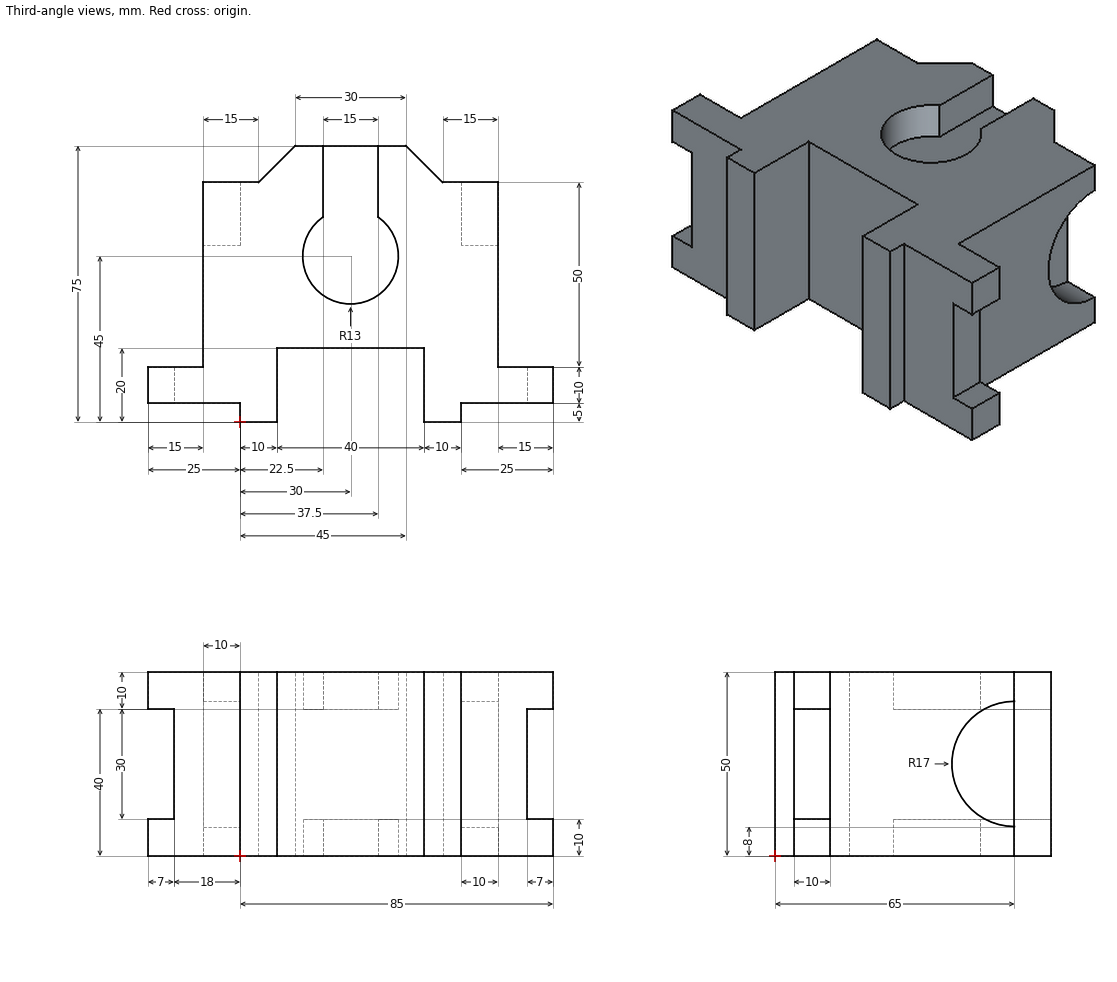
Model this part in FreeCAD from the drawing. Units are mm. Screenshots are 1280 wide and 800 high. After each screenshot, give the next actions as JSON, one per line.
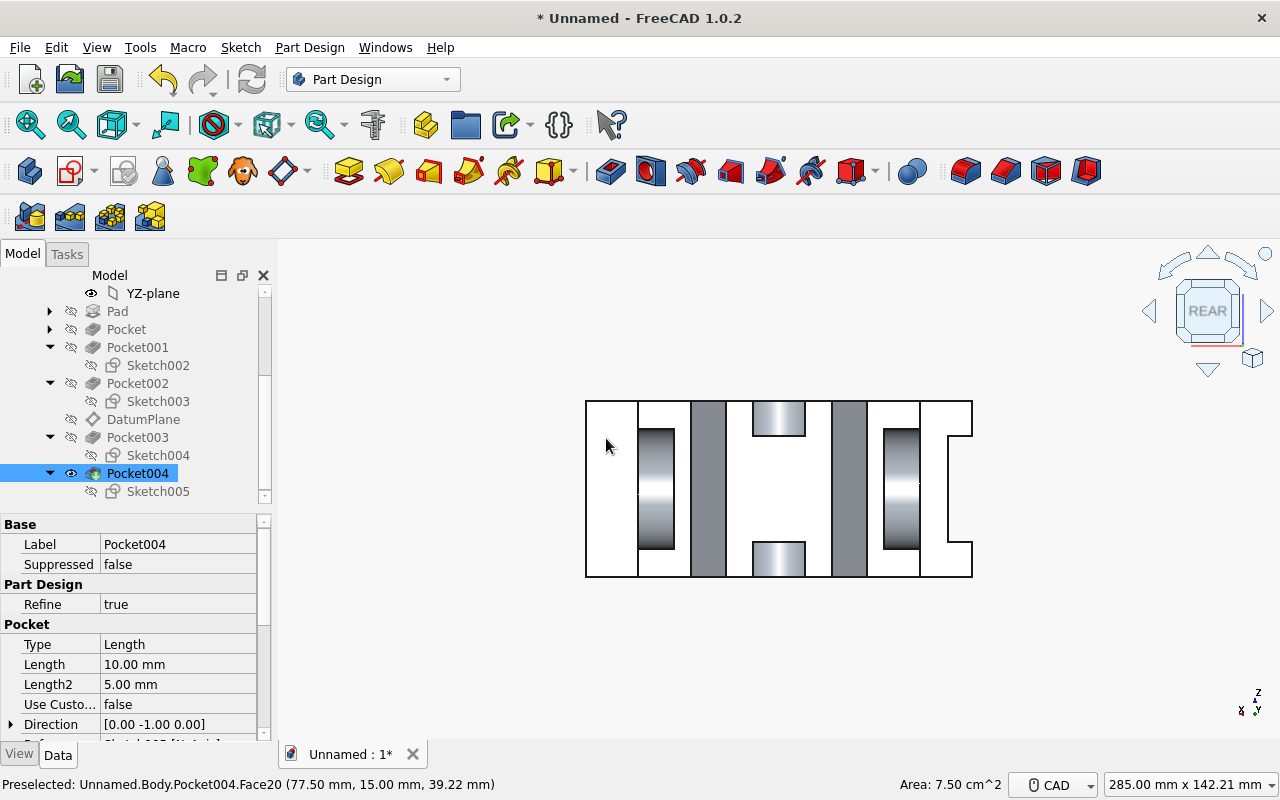
{"action": "left_click", "coordinate": [70, 172]}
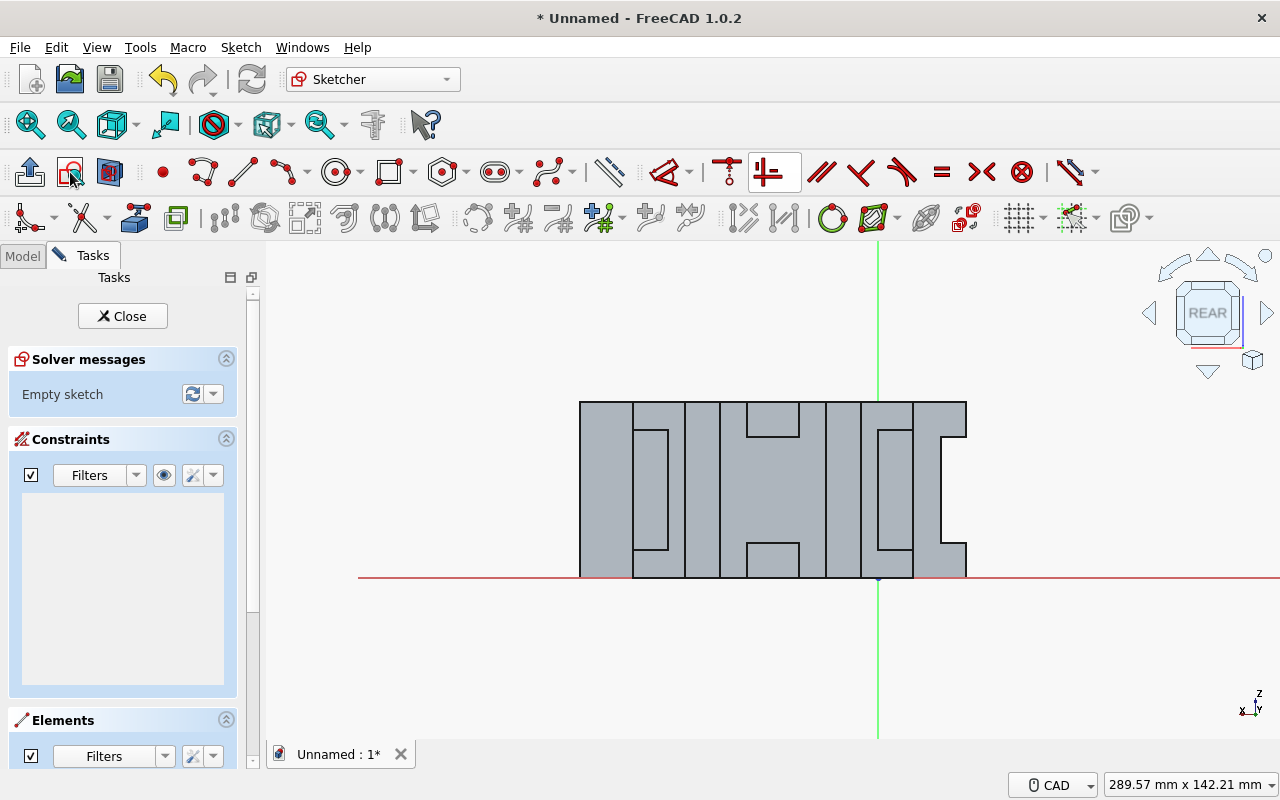
{"action": "scroll", "coordinate": [528, 490], "scroll_direction": "up", "scroll_amount": 5}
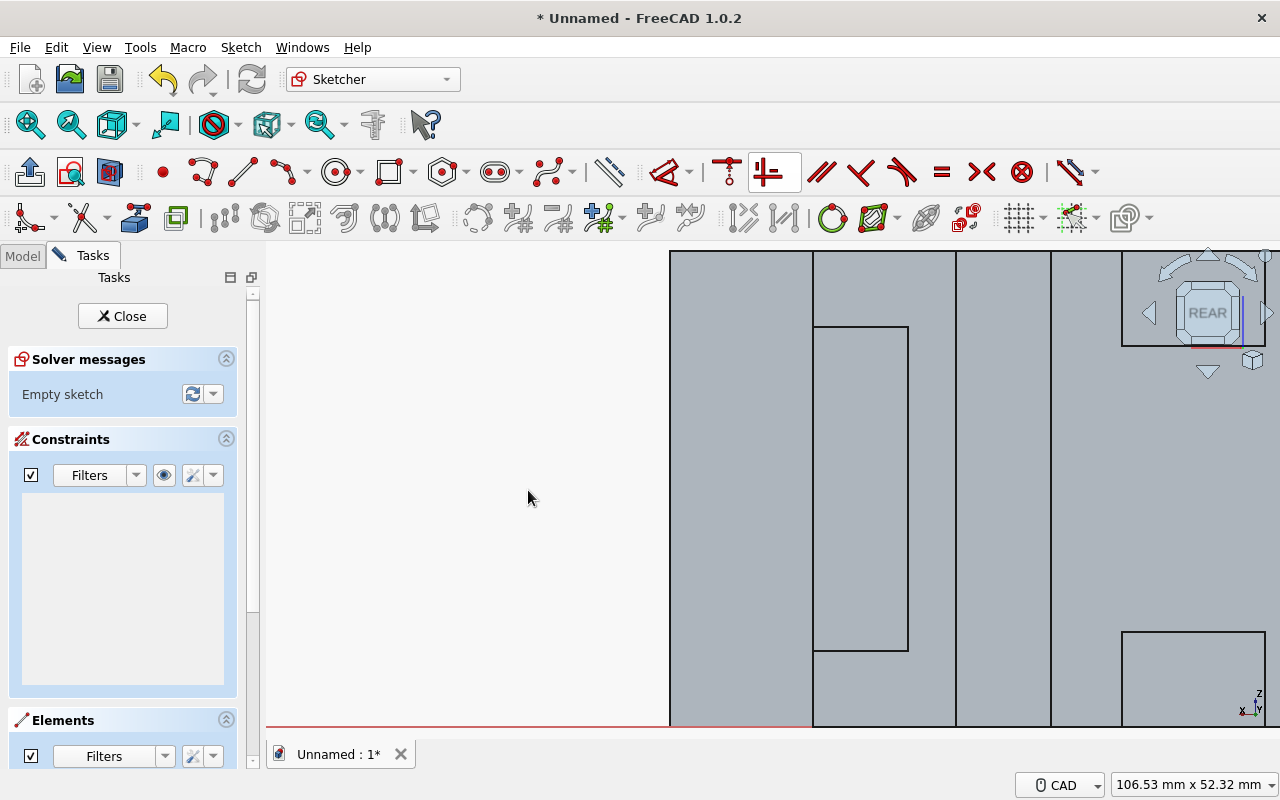
{"action": "left_click", "coordinate": [390, 172]}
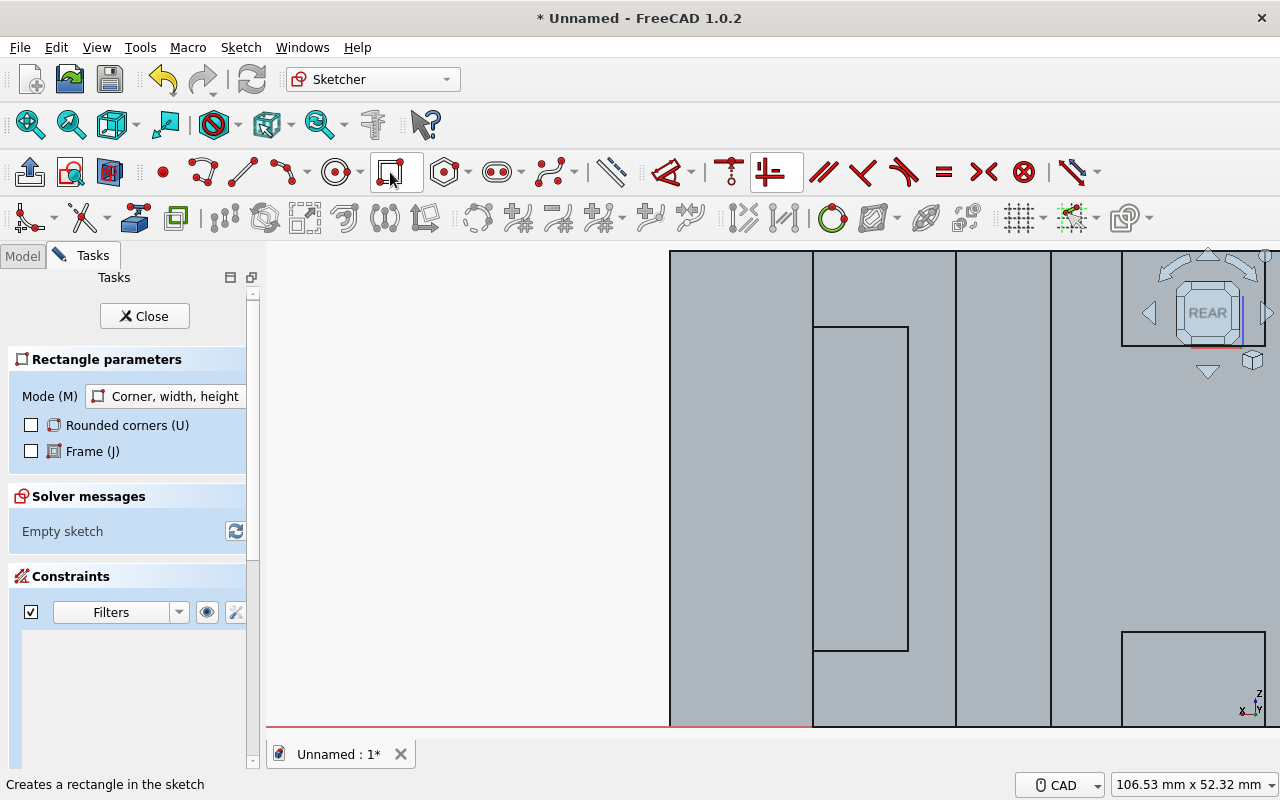
{"action": "left_click", "coordinate": [670, 346]}
{"action": "left_click", "coordinate": [737, 632]}
{"action": "key", "text": "Escape"}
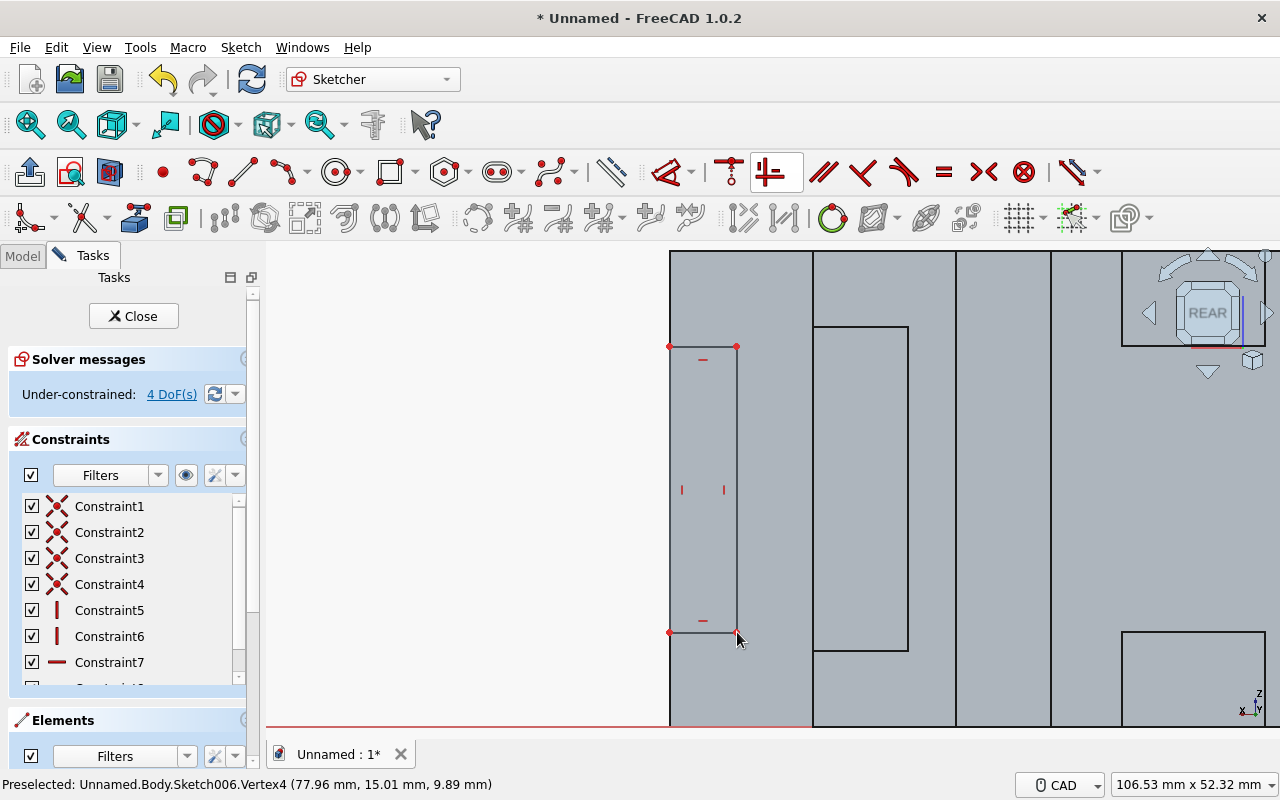
{"action": "left_click", "coordinate": [666, 172]}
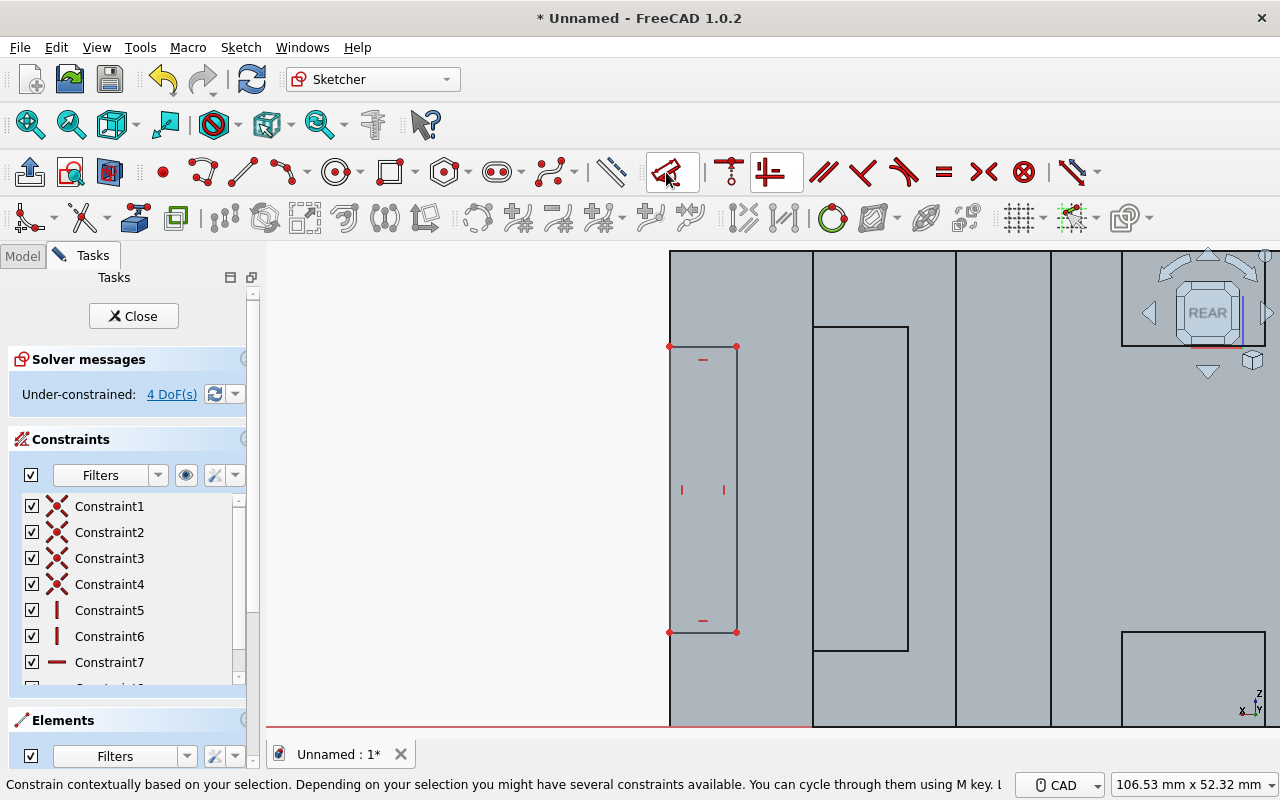
{"action": "left_click", "coordinate": [690, 633]}
{"action": "left_click", "coordinate": [704, 667]}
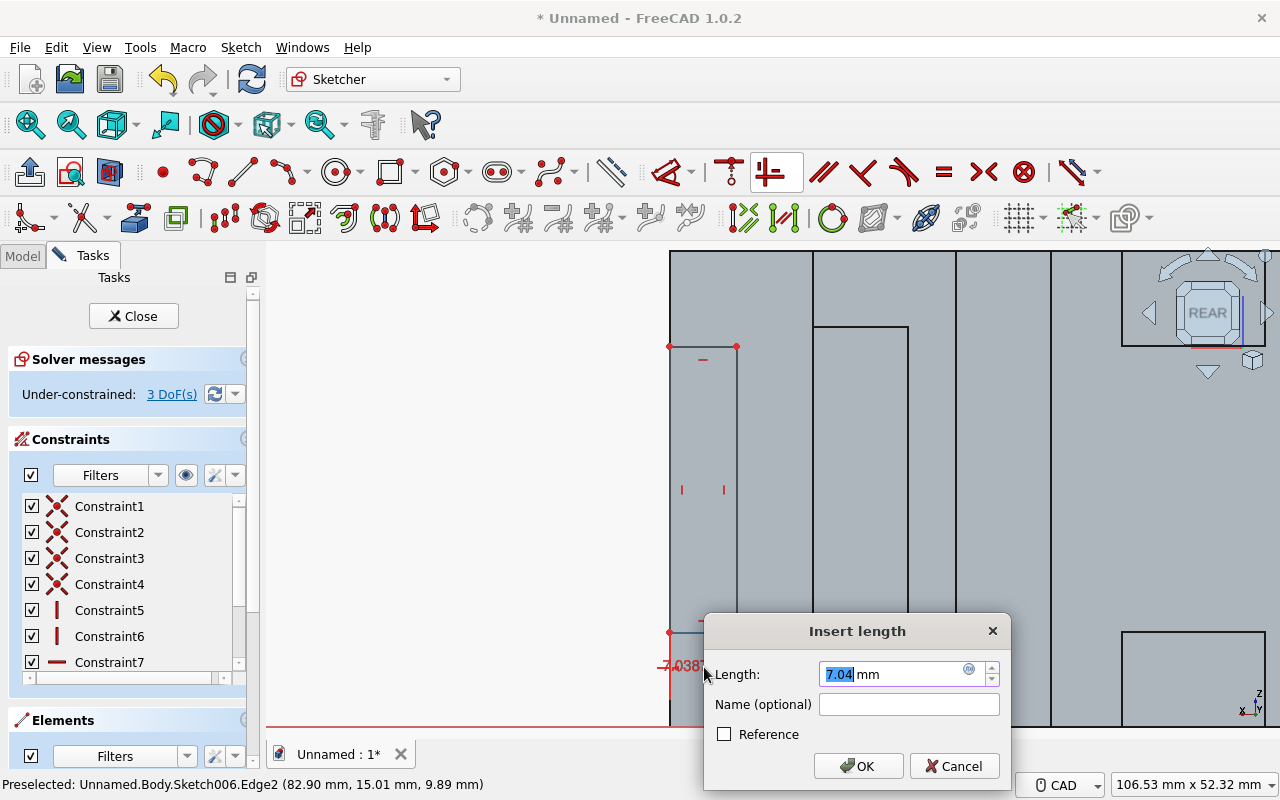
{"action": "type", "text": "7"}
{"action": "key", "text": "Return"}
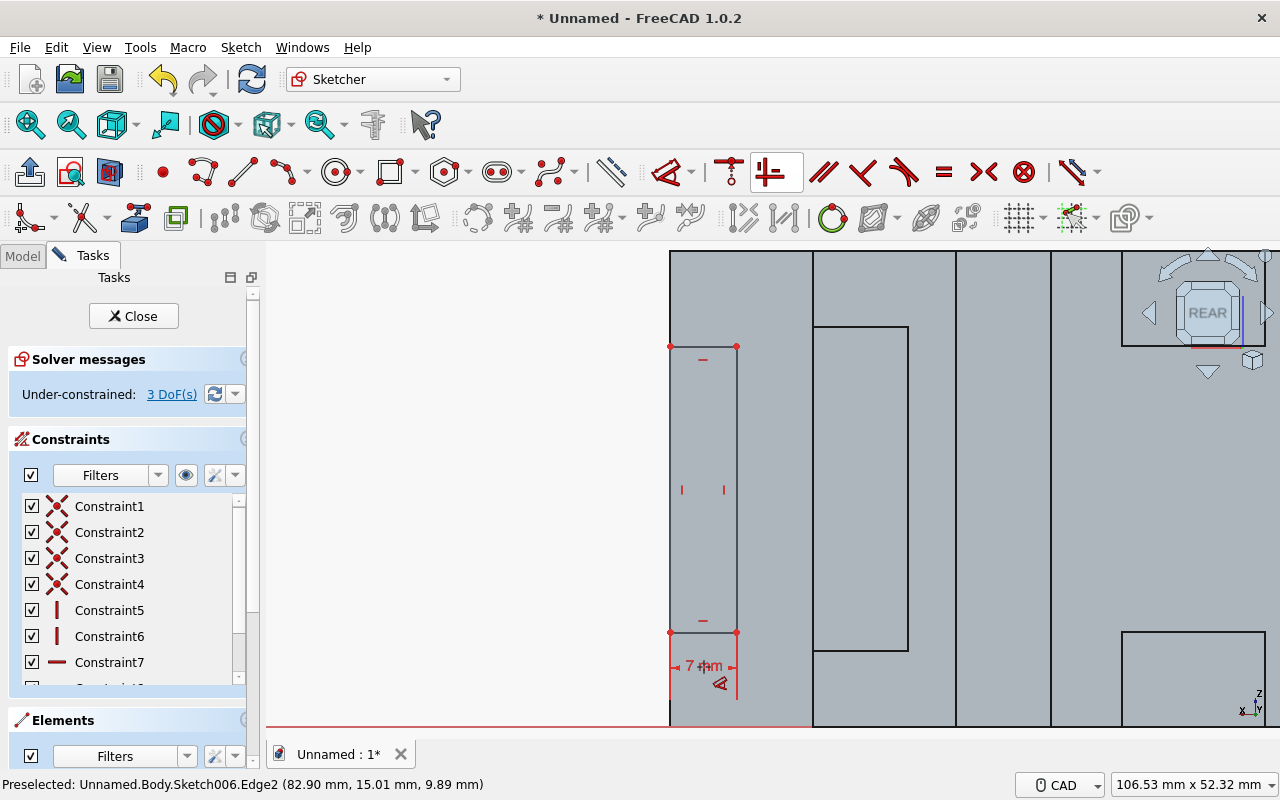
{"action": "left_click", "coordinate": [670, 433]}
{"action": "left_click", "coordinate": [636, 490]}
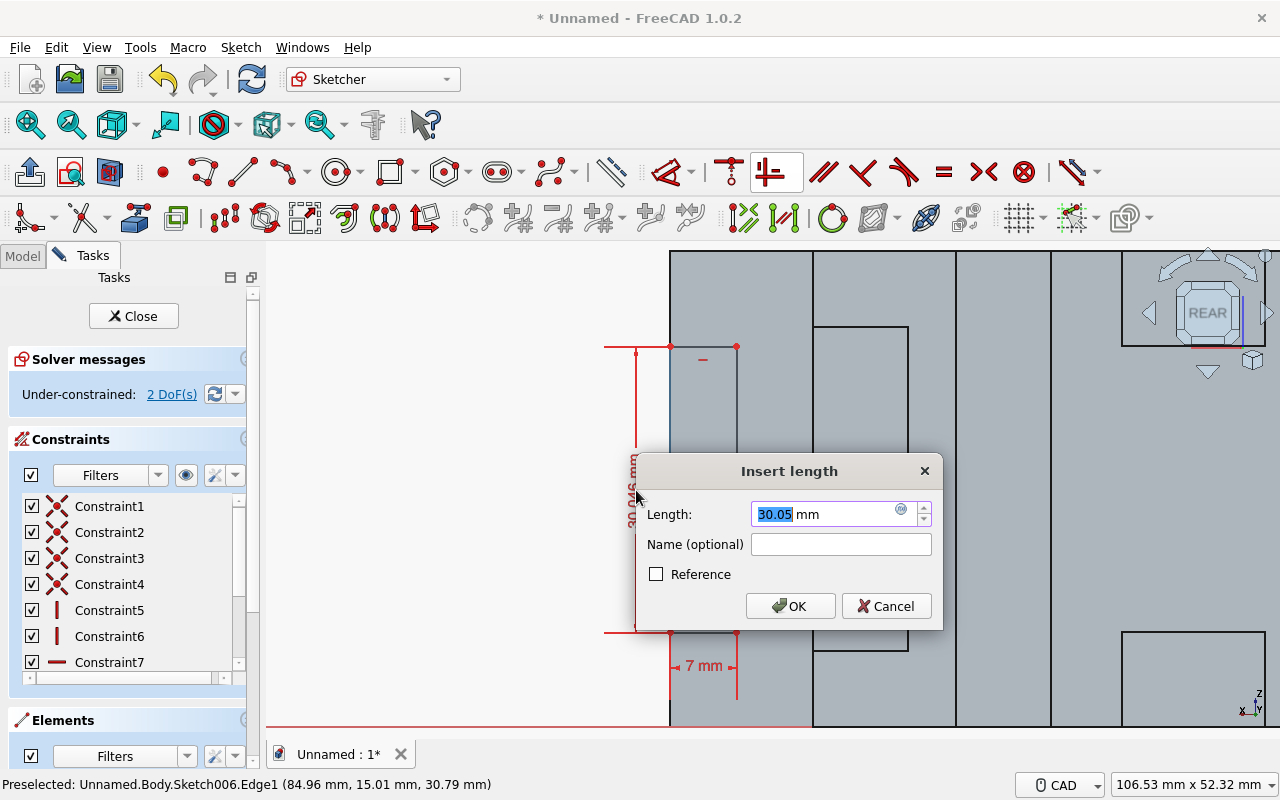
{"action": "type", "text": "30"}
{"action": "key", "text": "Return"}